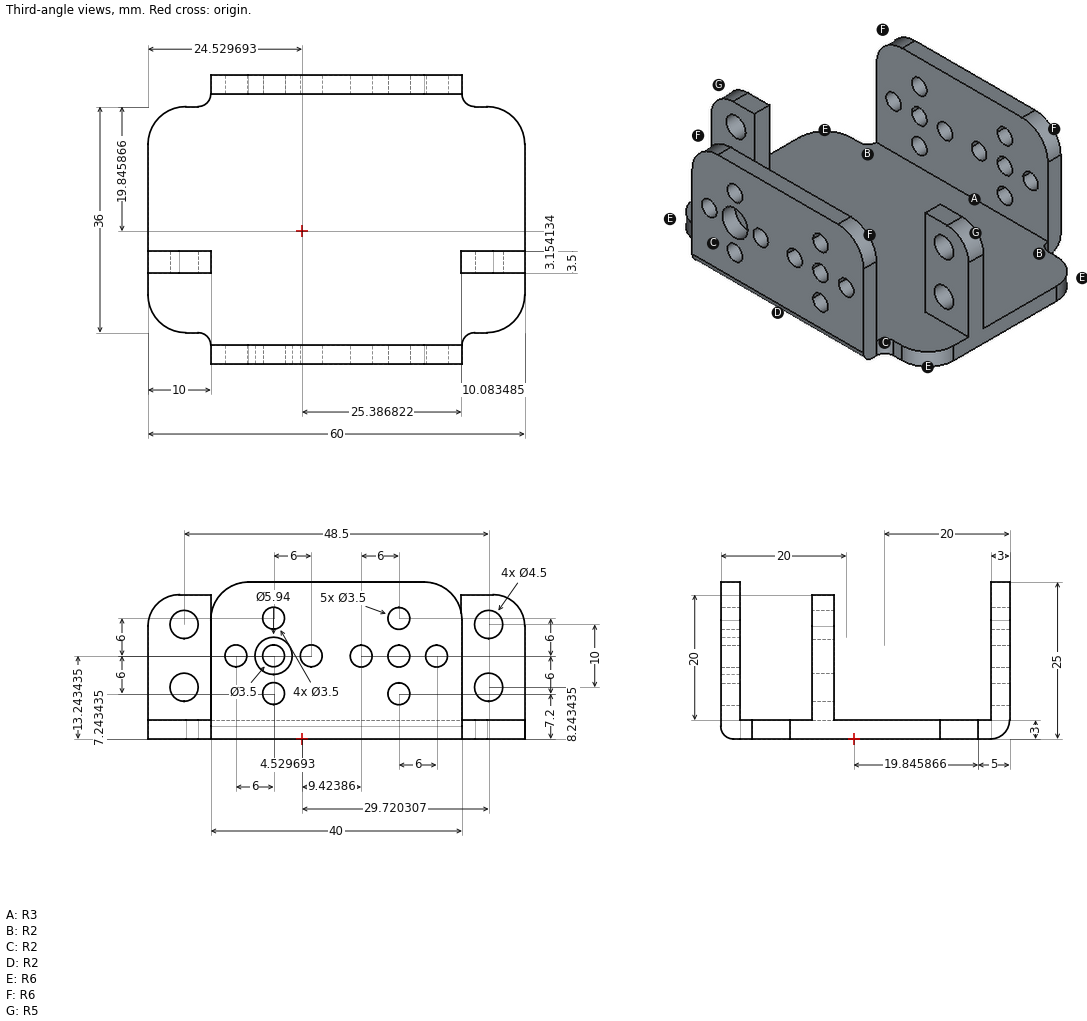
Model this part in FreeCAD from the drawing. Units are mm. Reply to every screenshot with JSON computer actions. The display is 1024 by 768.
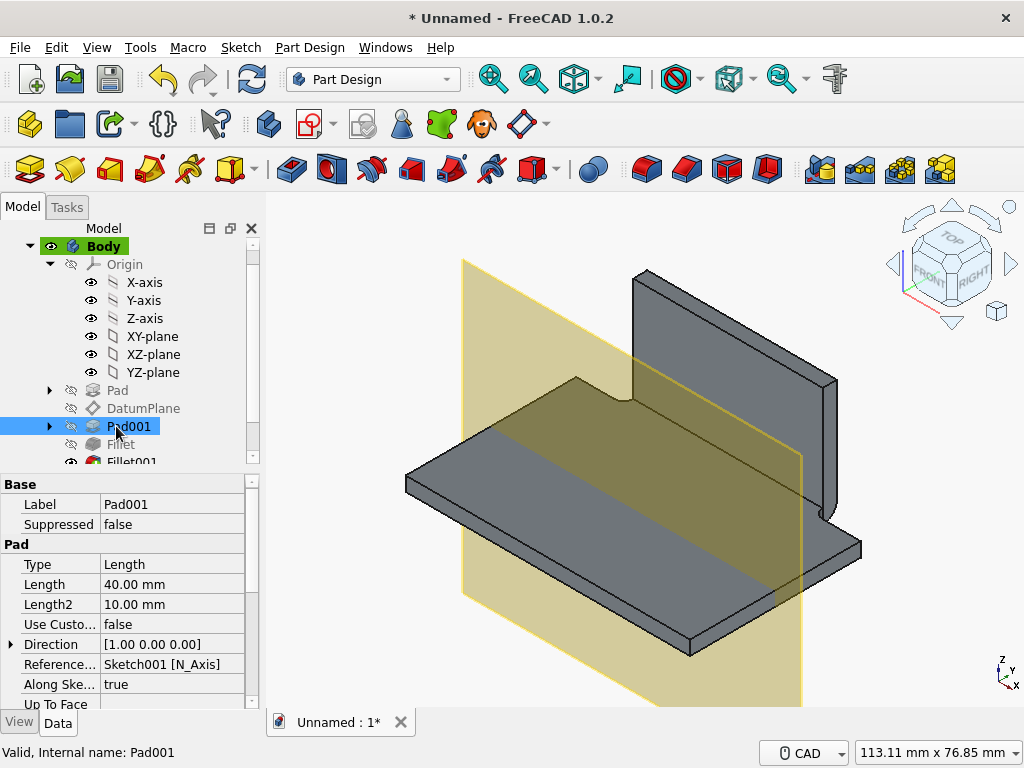
{"action": "left_click", "coordinate": [820, 170]}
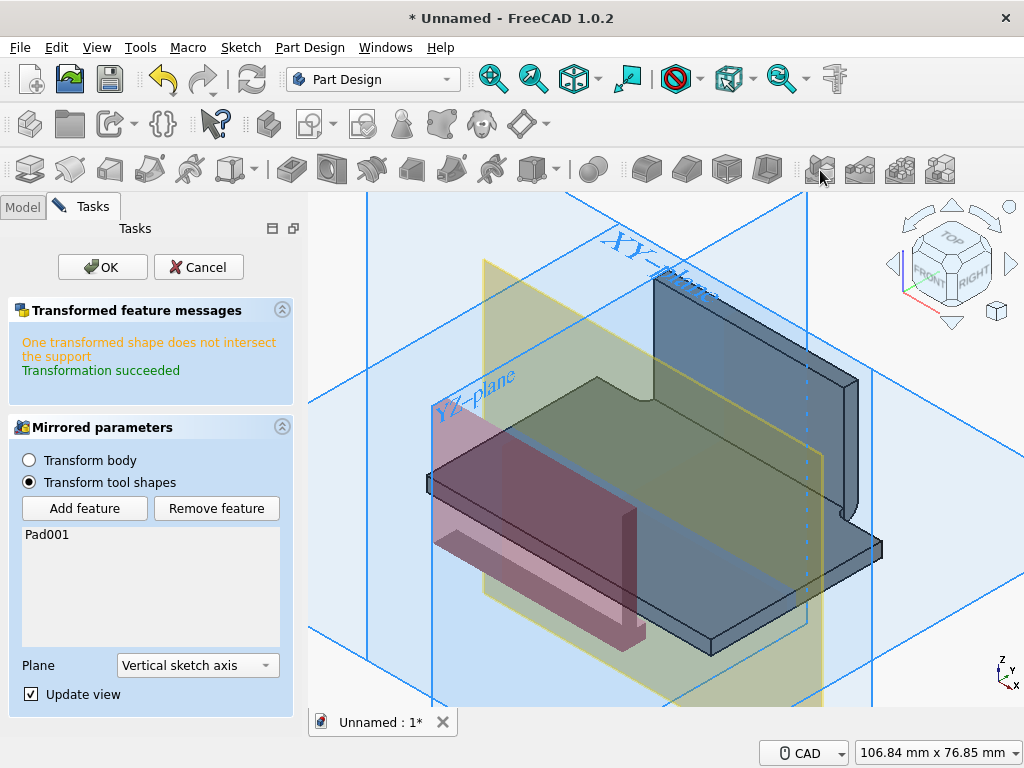
{"action": "left_click", "coordinate": [198, 666]}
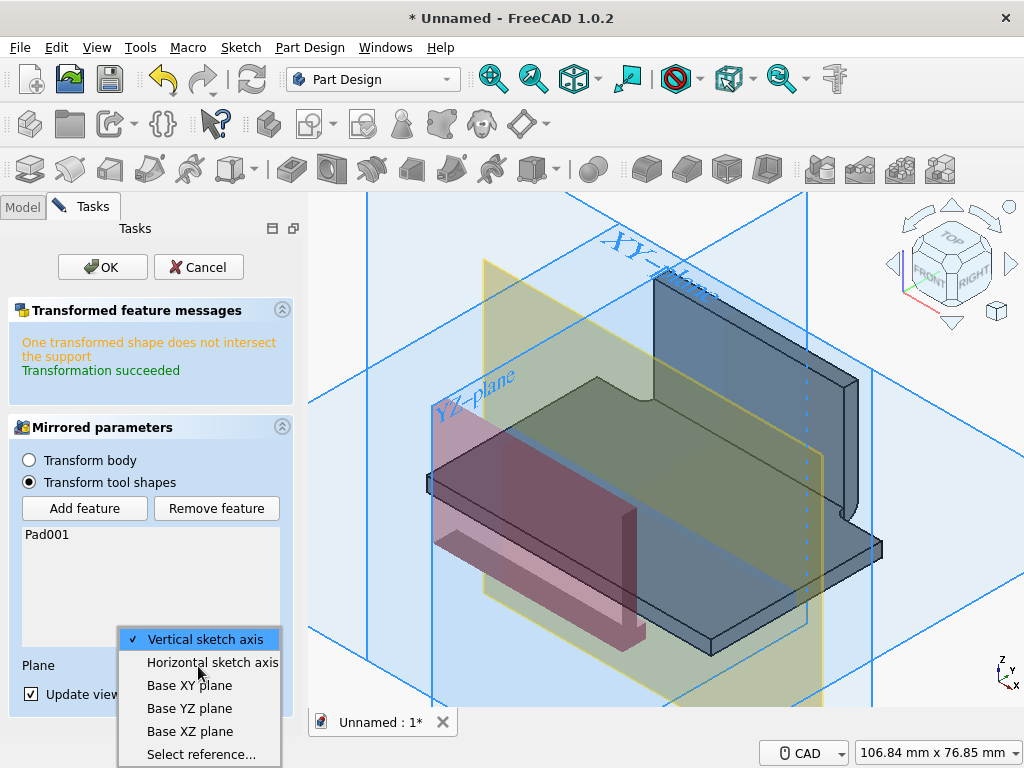
{"action": "left_click", "coordinate": [198, 754]}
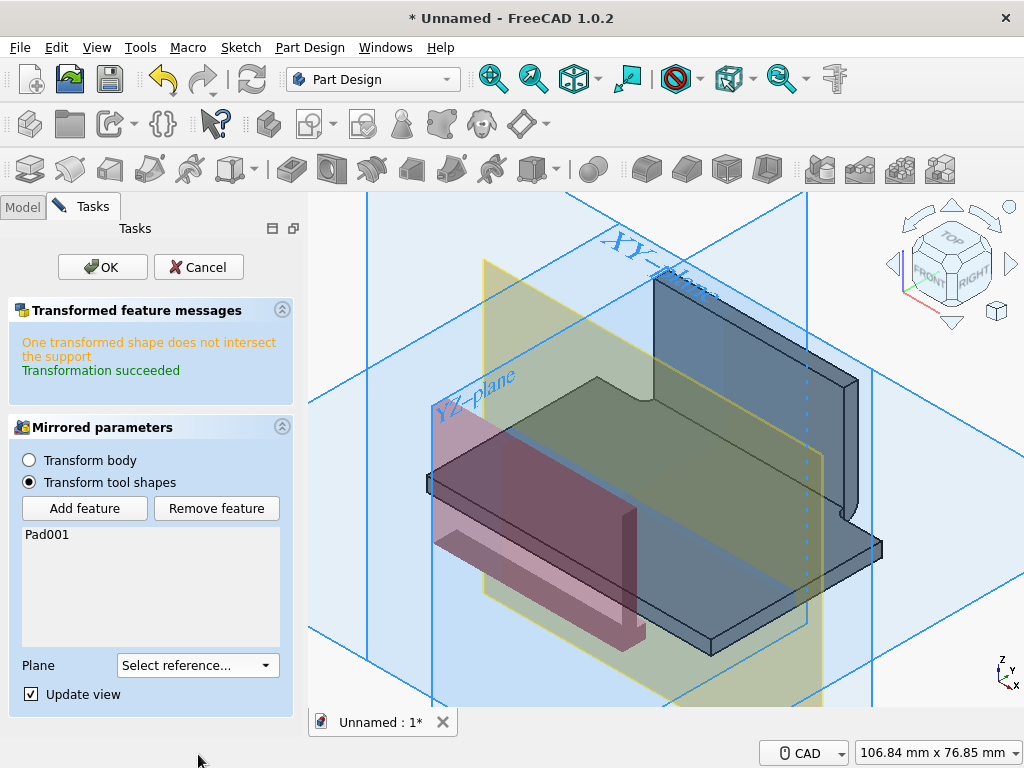
{"action": "left_click", "coordinate": [23, 206]}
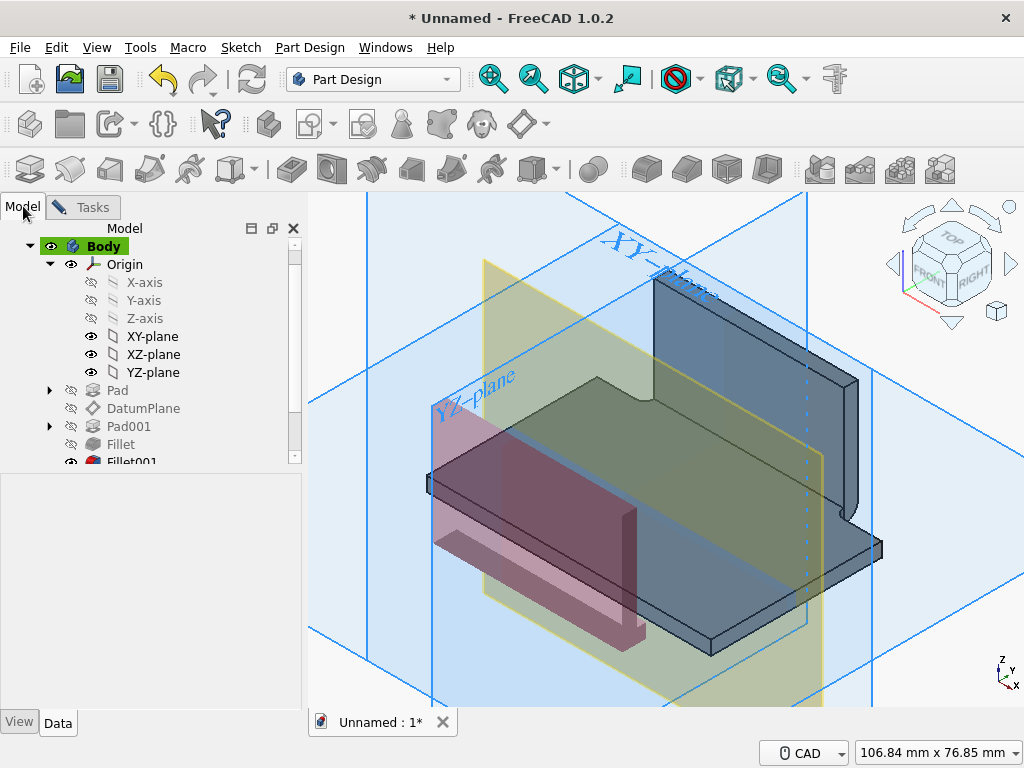
{"action": "scroll", "coordinate": [120, 350], "scroll_direction": "down", "scroll_amount": 3}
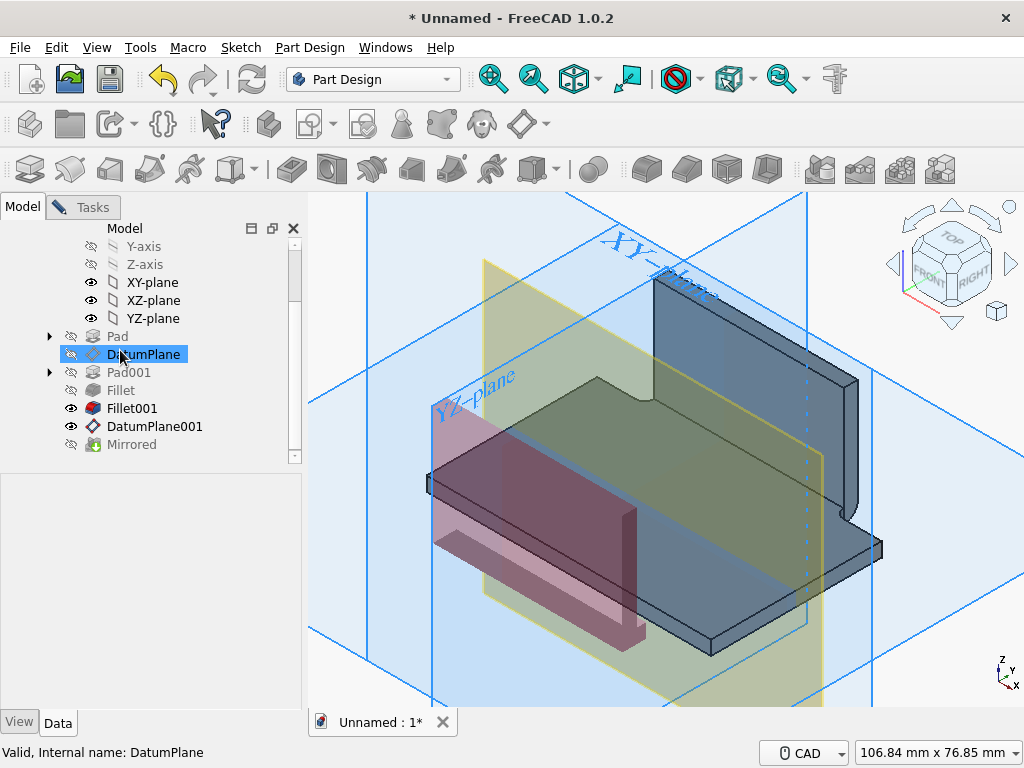
{"action": "left_click", "coordinate": [116, 426]}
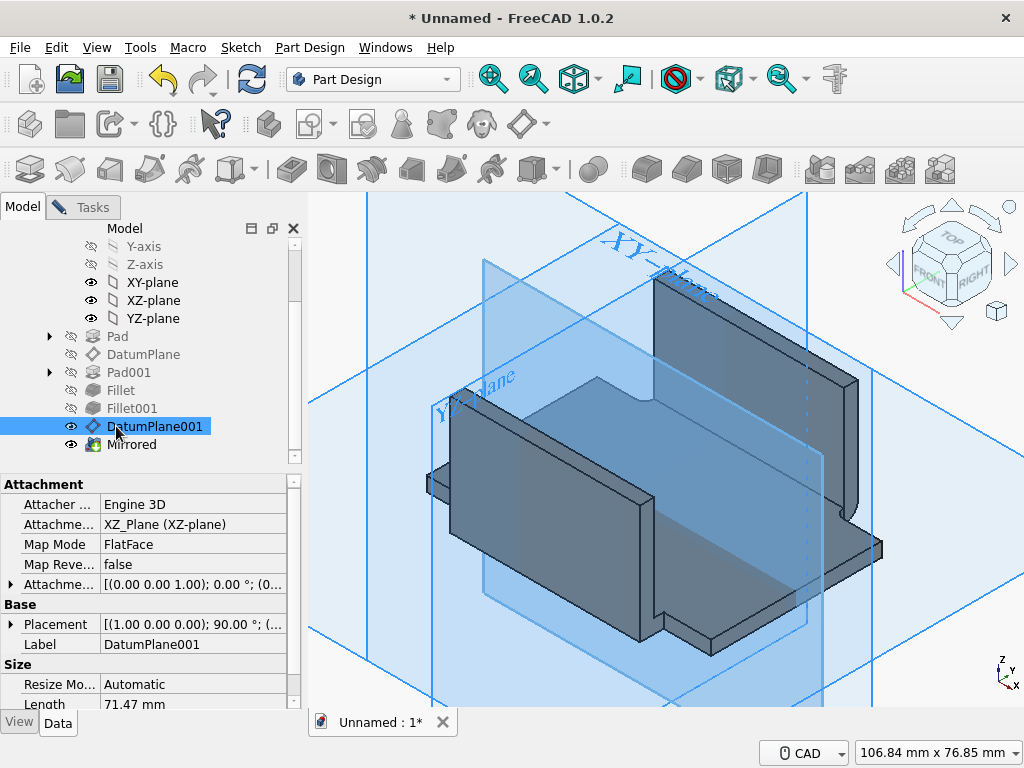
{"action": "left_click", "coordinate": [84, 206]}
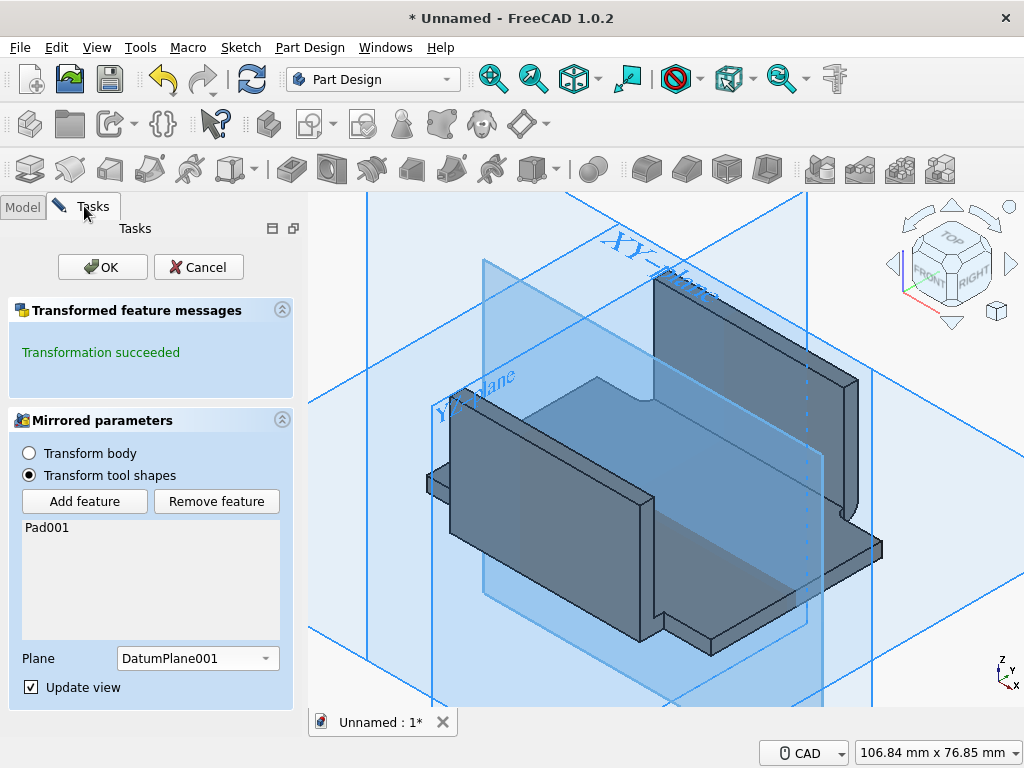
{"action": "left_click", "coordinate": [103, 267]}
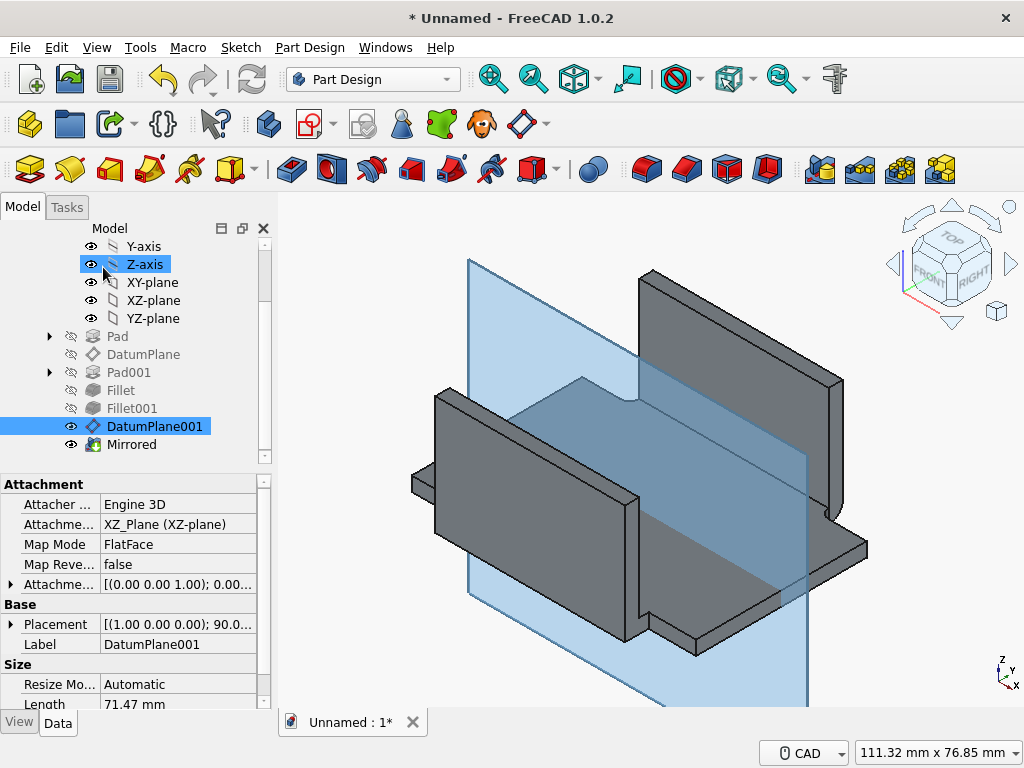
{"action": "left_click", "coordinate": [116, 426]}
{"action": "key", "text": "space"}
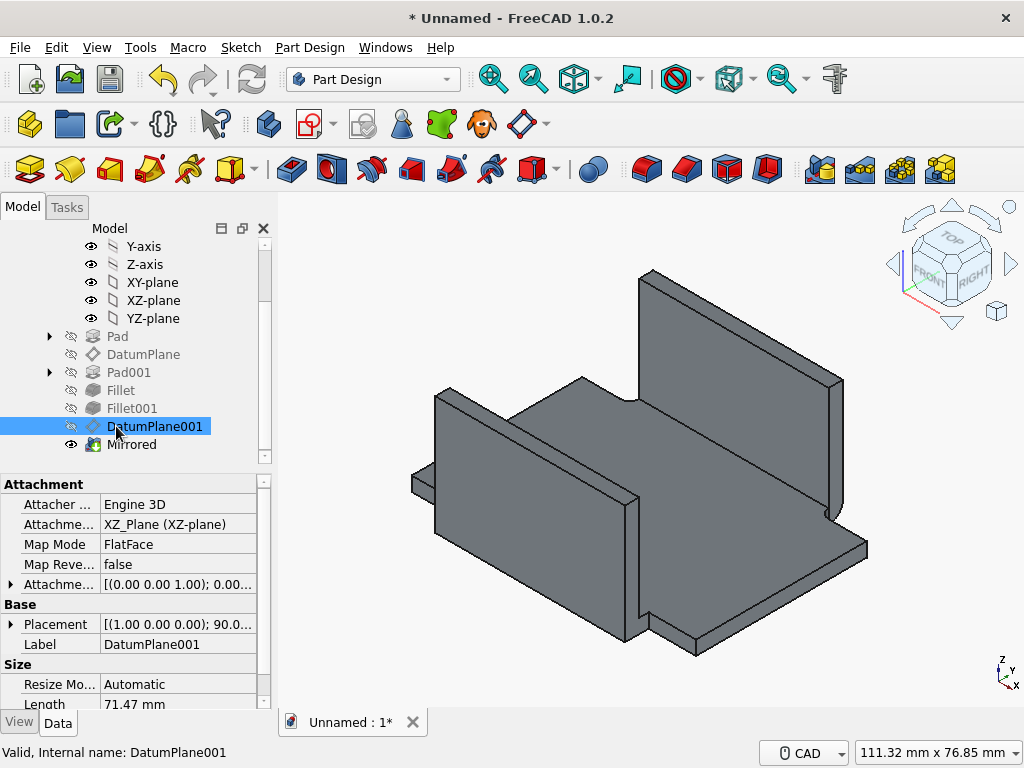
{"action": "scroll", "coordinate": [649, 619], "scroll_direction": "up", "scroll_amount": 4}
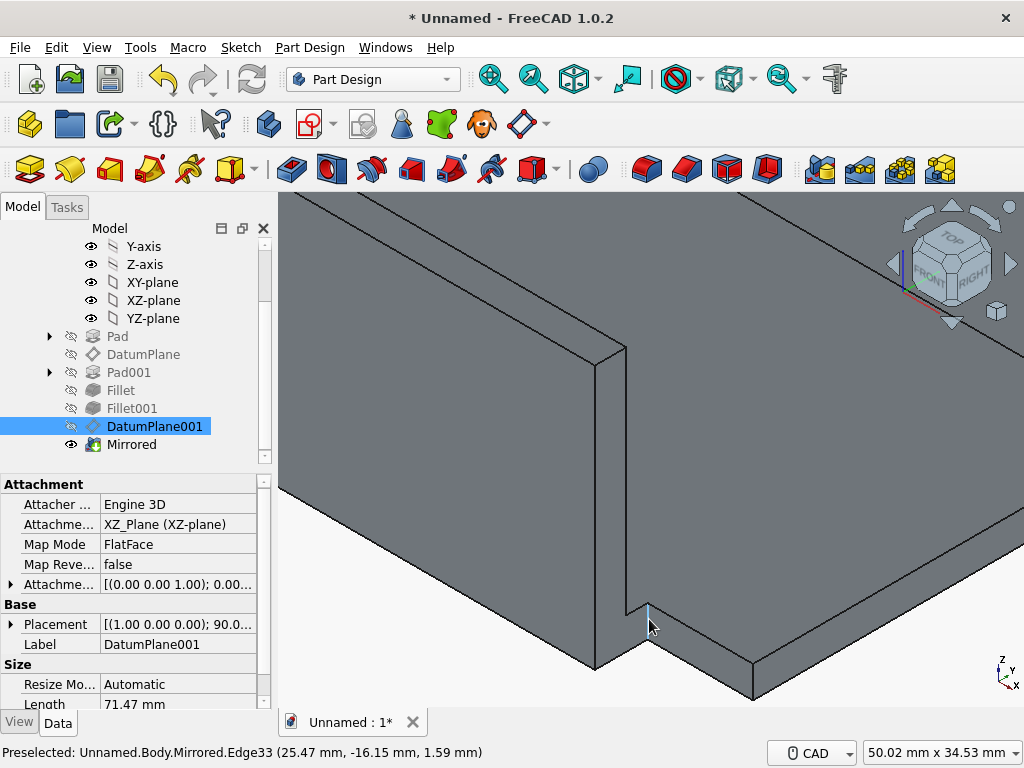
{"action": "left_click", "coordinate": [494, 80]}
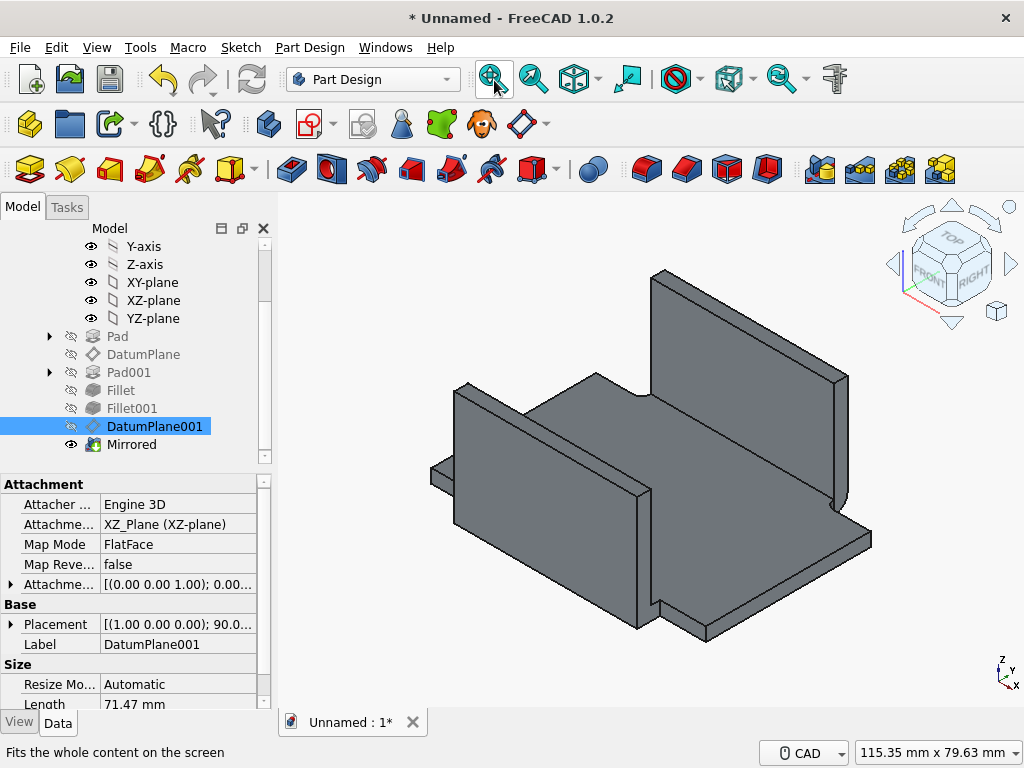
{"action": "key", "text": "2"}